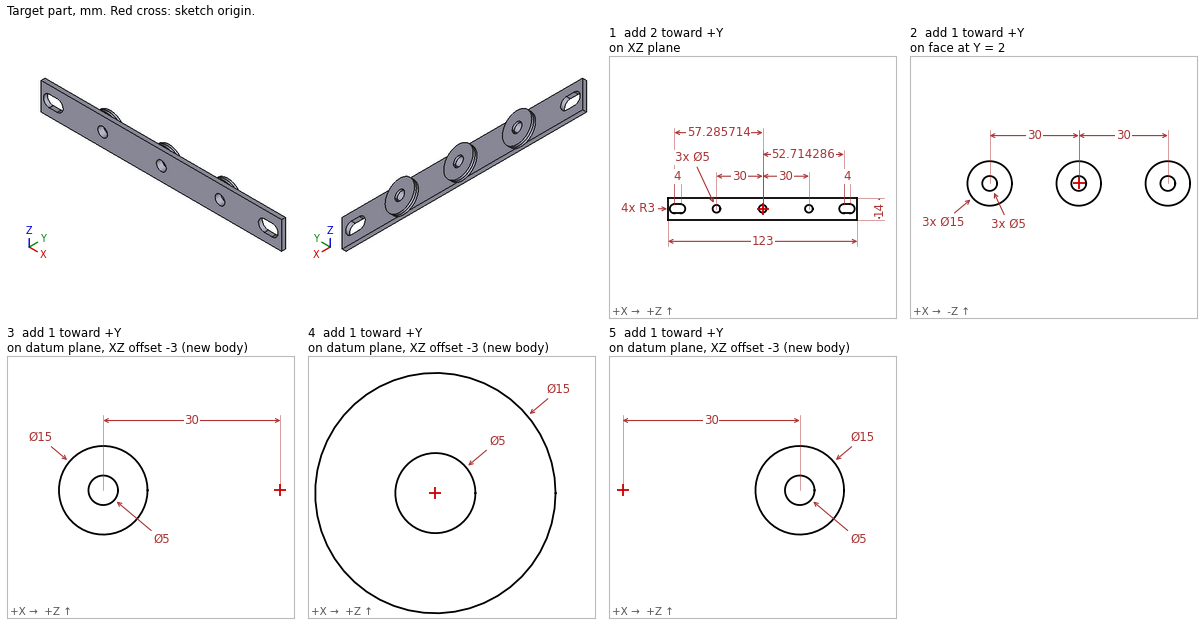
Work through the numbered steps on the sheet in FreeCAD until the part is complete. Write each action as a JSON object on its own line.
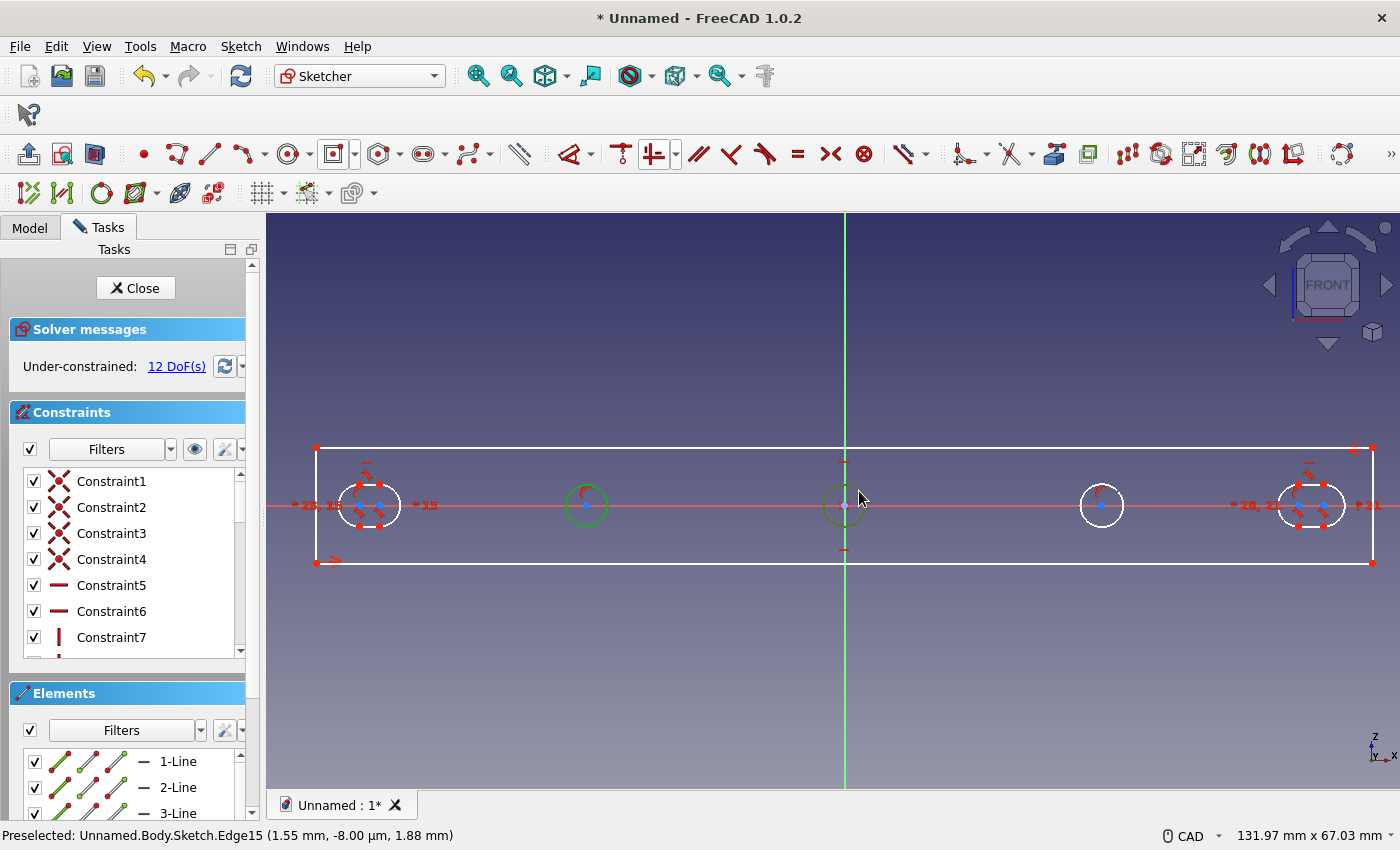
{"action": "left_click", "coordinate": [1117, 490]}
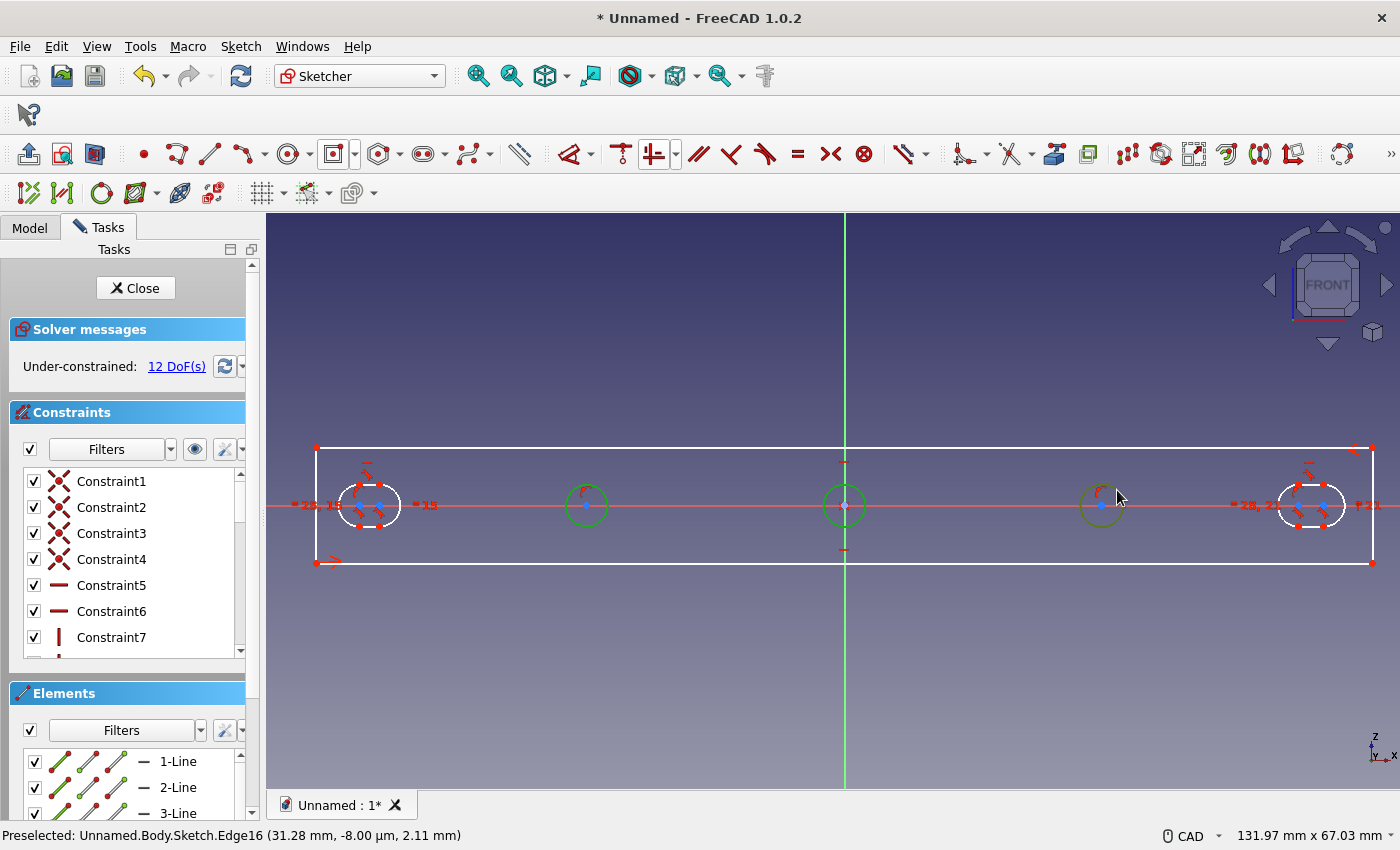
{"action": "left_click", "coordinate": [798, 154]}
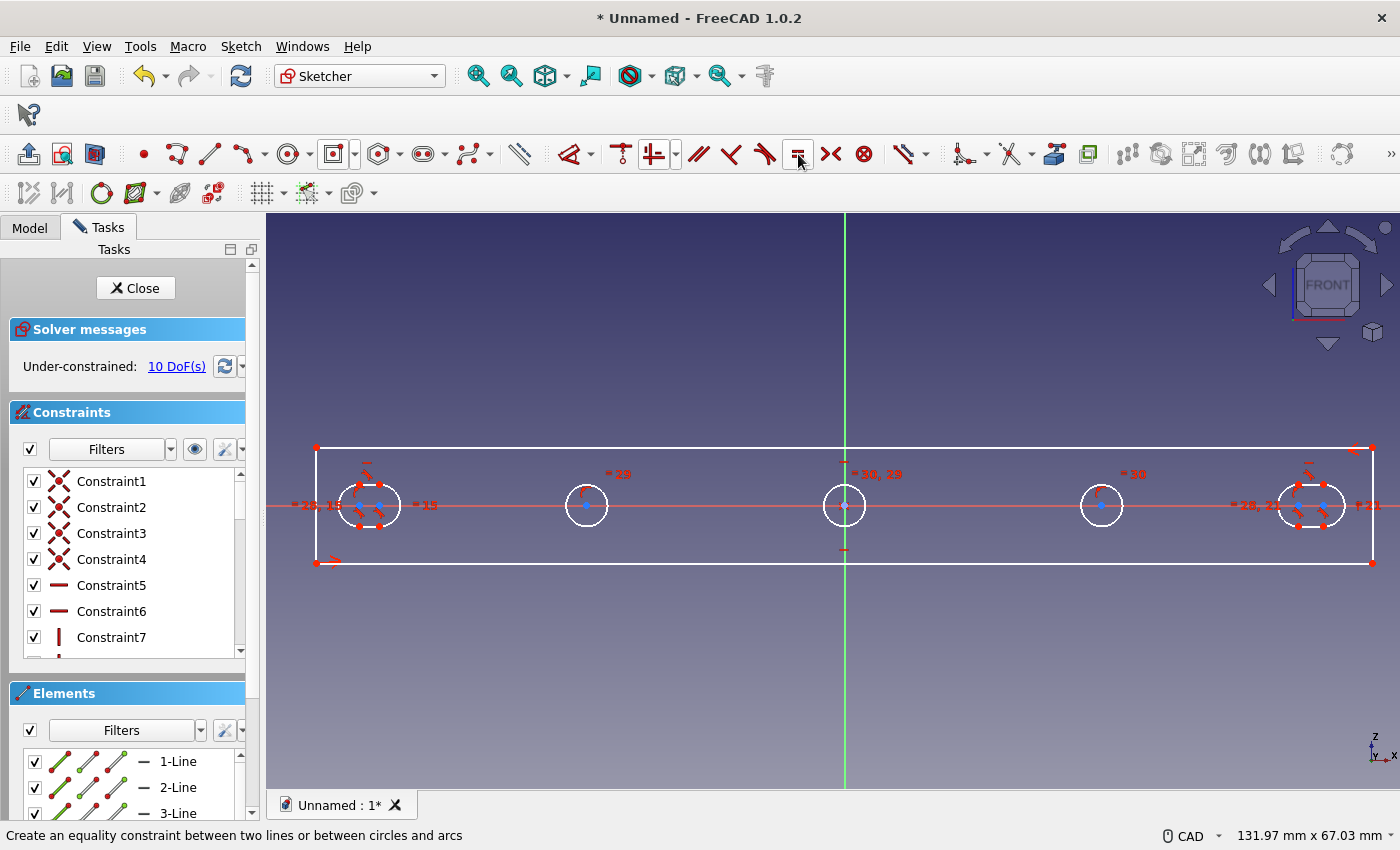
{"action": "scroll", "coordinate": [343, 493], "scroll_direction": "up", "scroll_amount": 3}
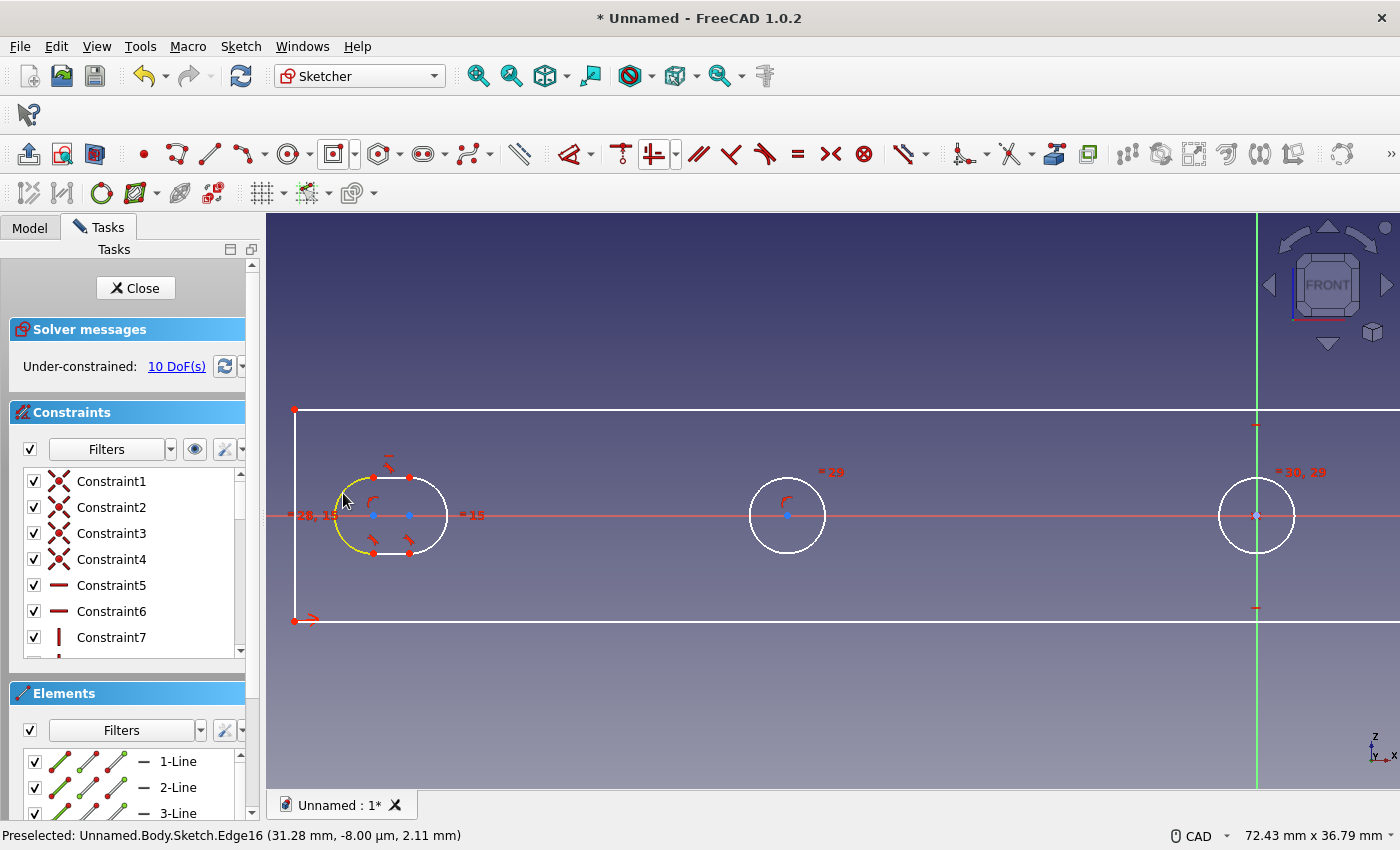
{"action": "left_click", "coordinate": [342, 493]}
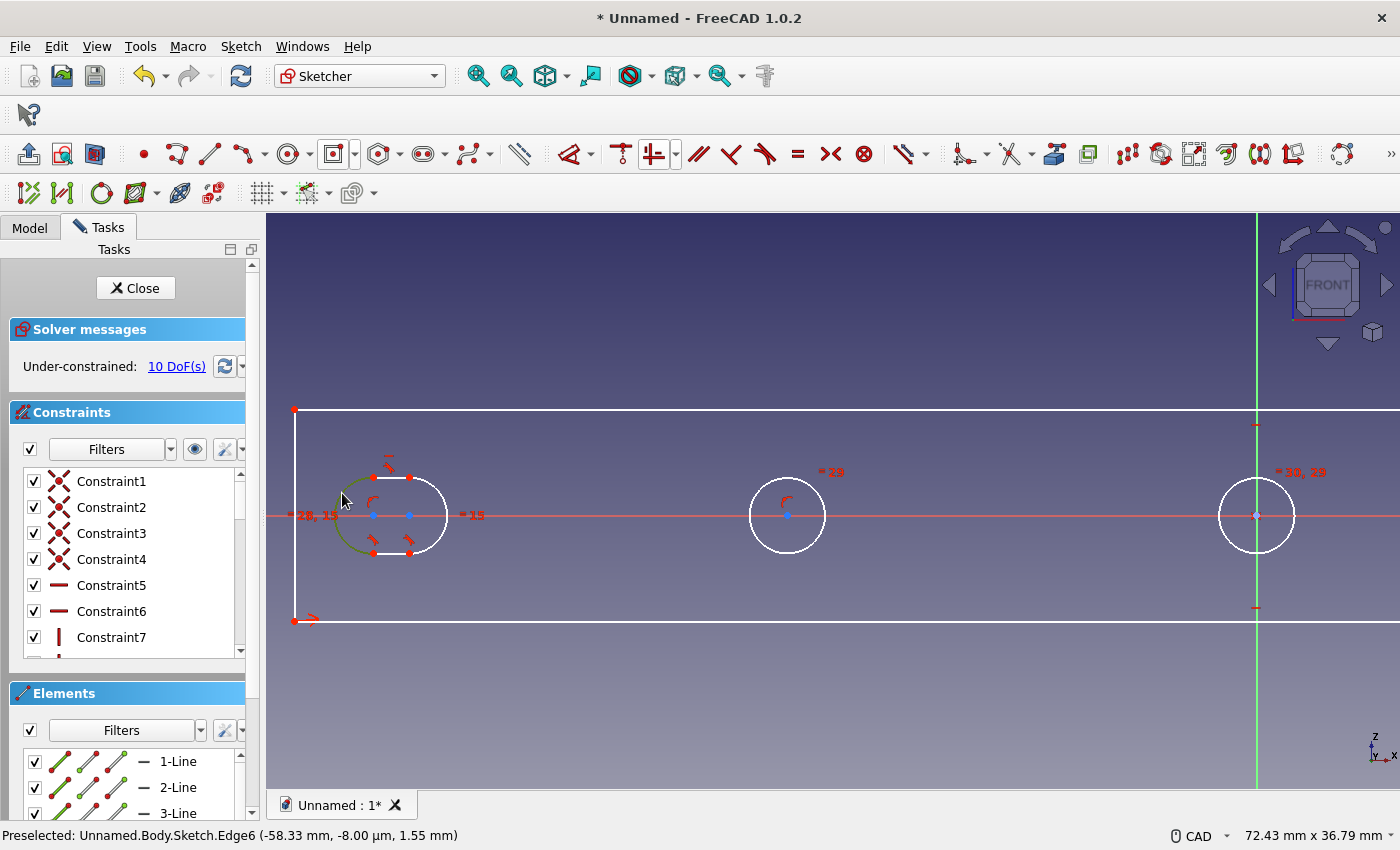
{"action": "left_click", "coordinate": [590, 154]}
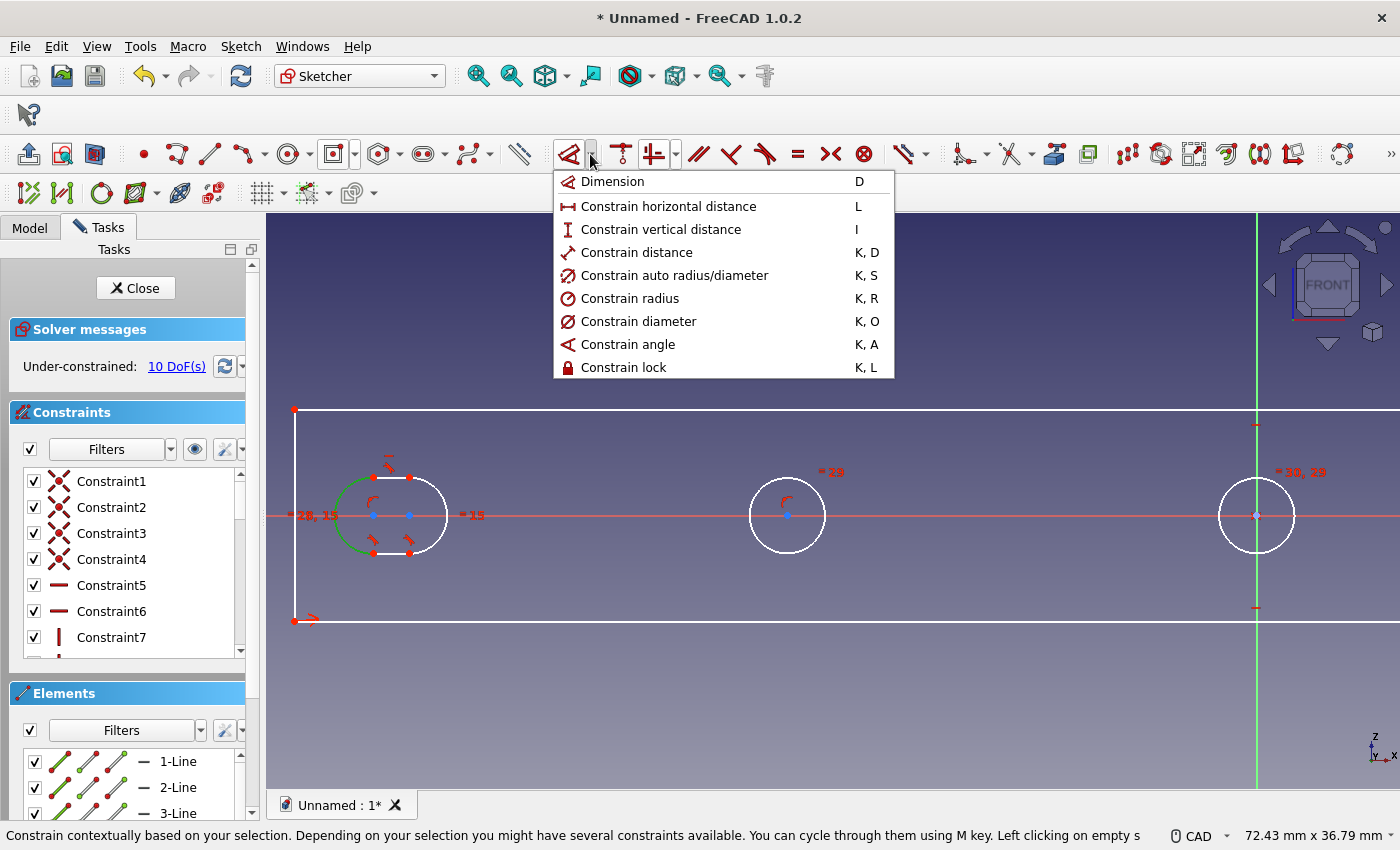
{"action": "left_click", "coordinate": [724, 298]}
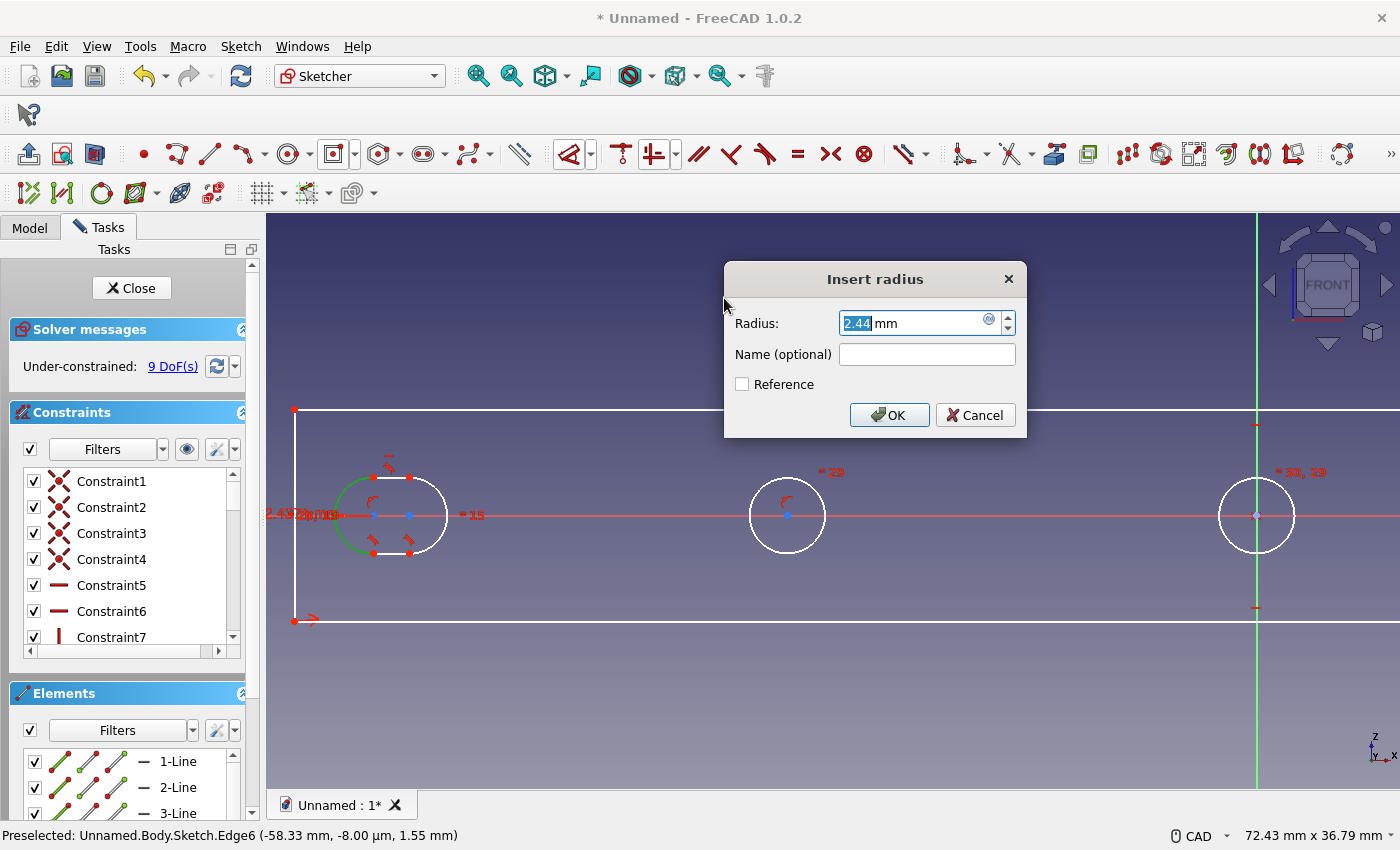
{"action": "type", "text": "3"}
{"action": "key", "text": "Return"}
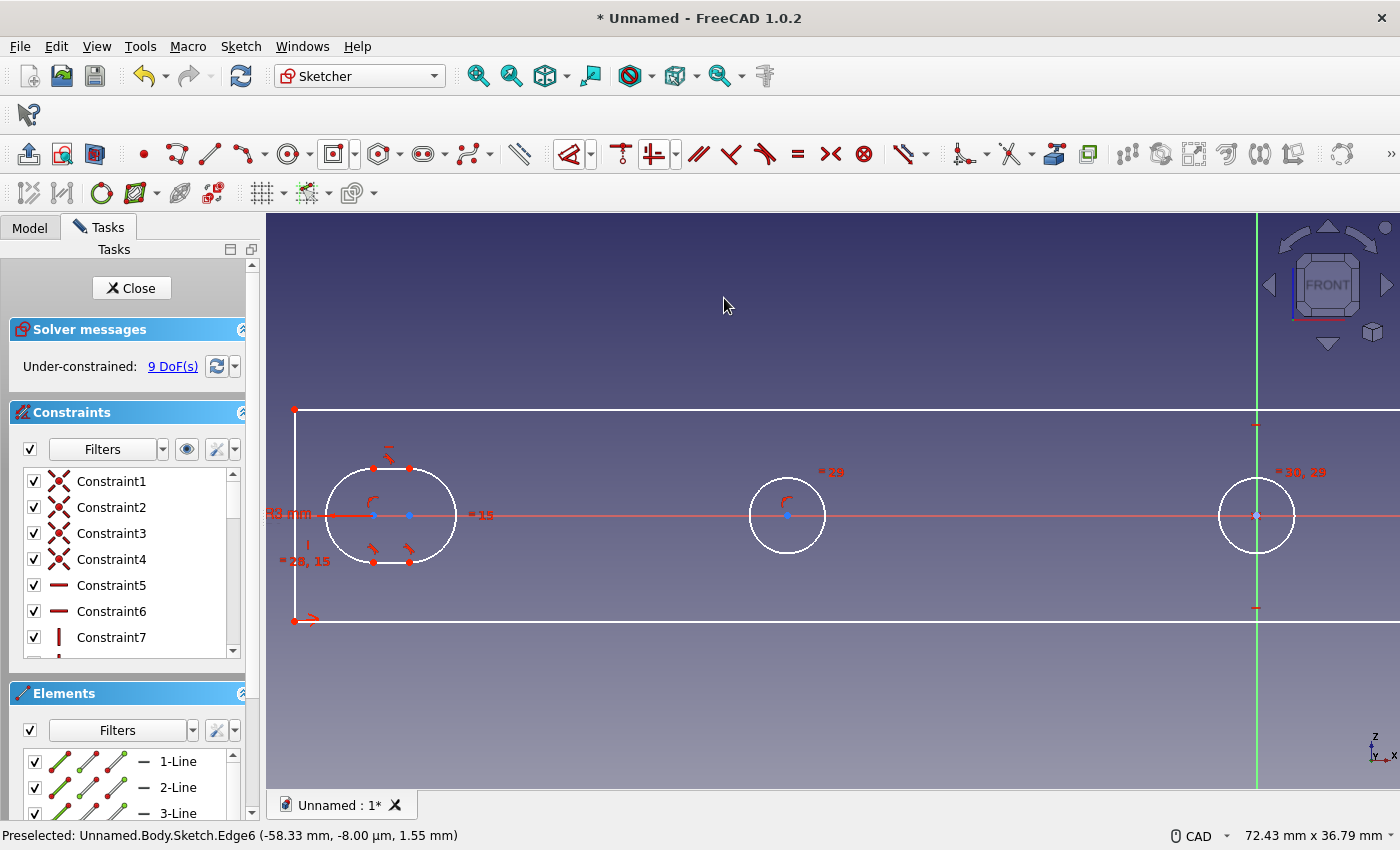
{"action": "left_click", "coordinate": [814, 489]}